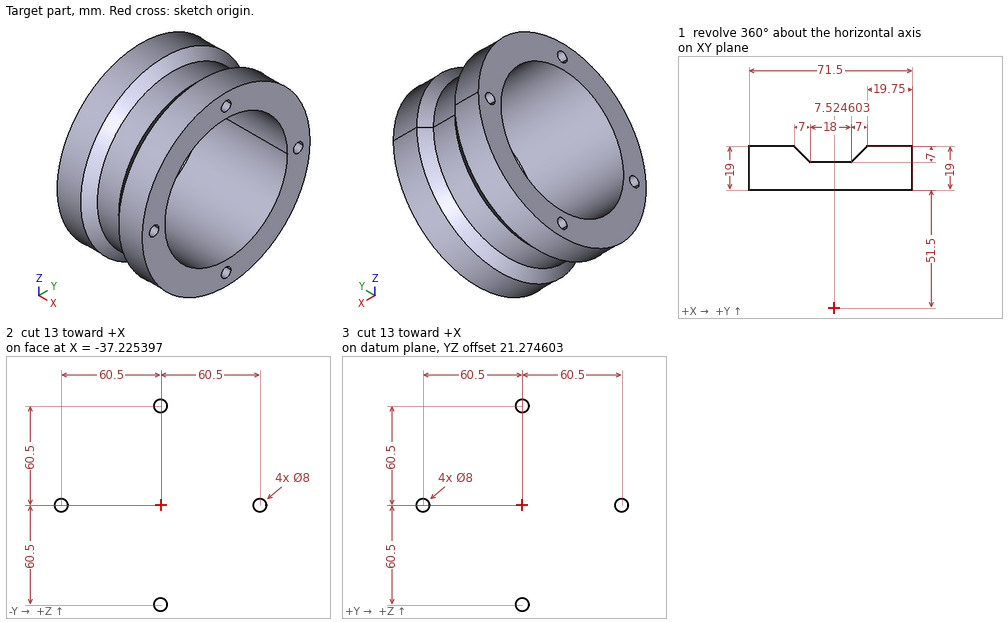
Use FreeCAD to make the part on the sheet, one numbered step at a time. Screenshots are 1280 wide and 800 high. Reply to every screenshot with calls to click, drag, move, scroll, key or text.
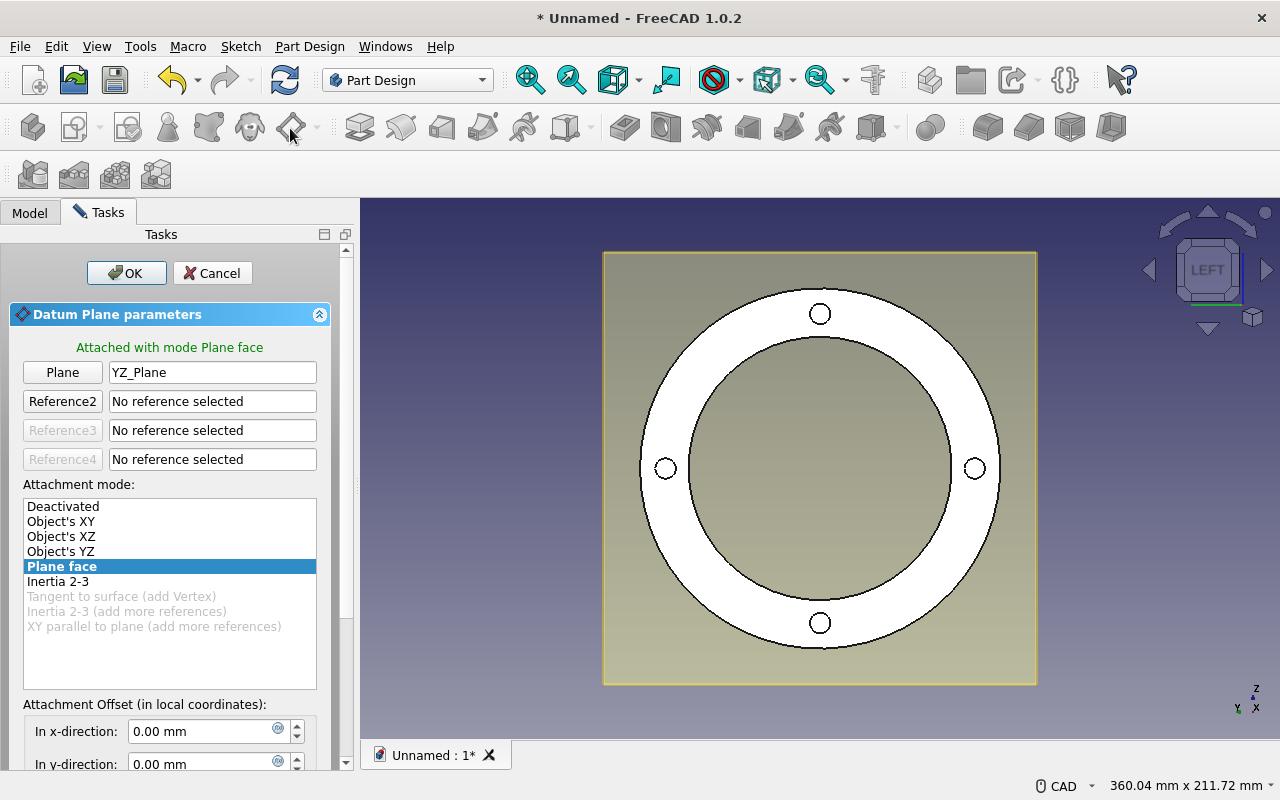
scroll(346, 507, down, 2)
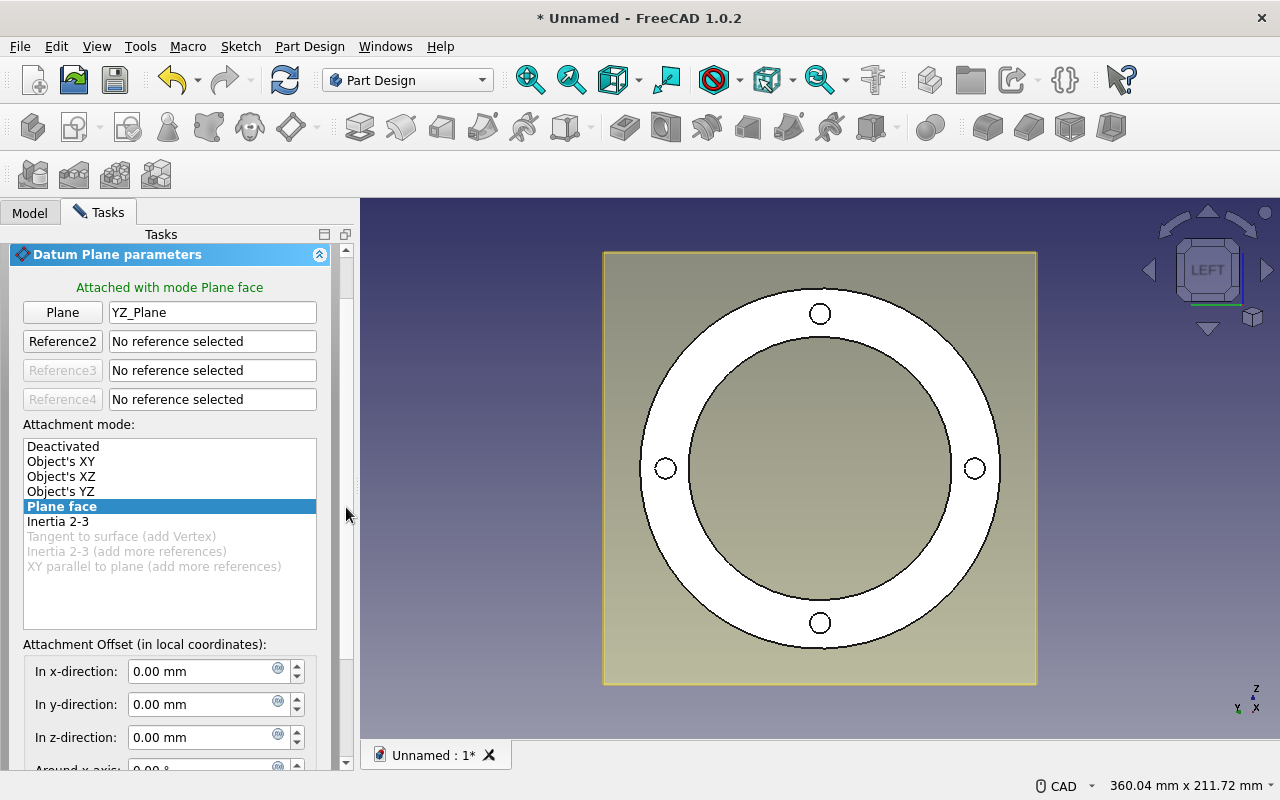
triple_click(210, 678)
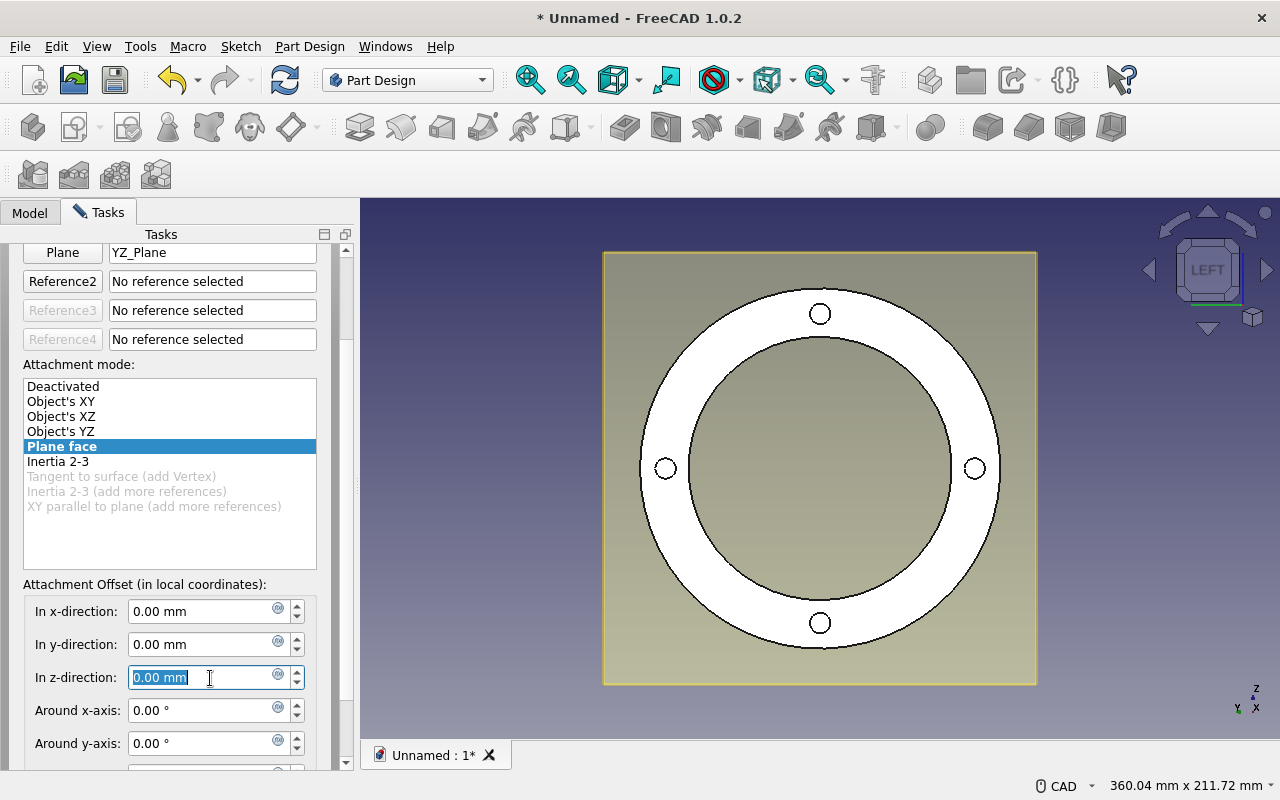
text(21.274603)
key(Tab)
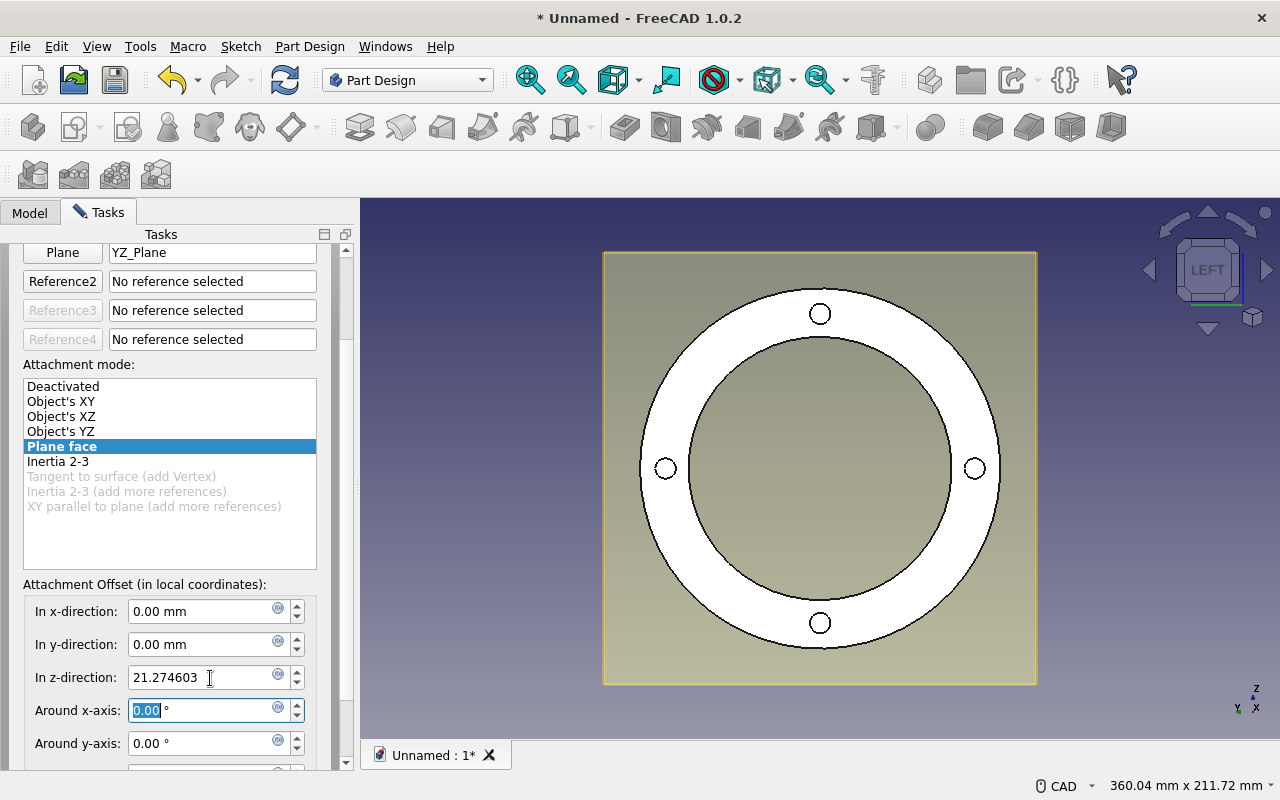
scroll(346, 507, up, 3)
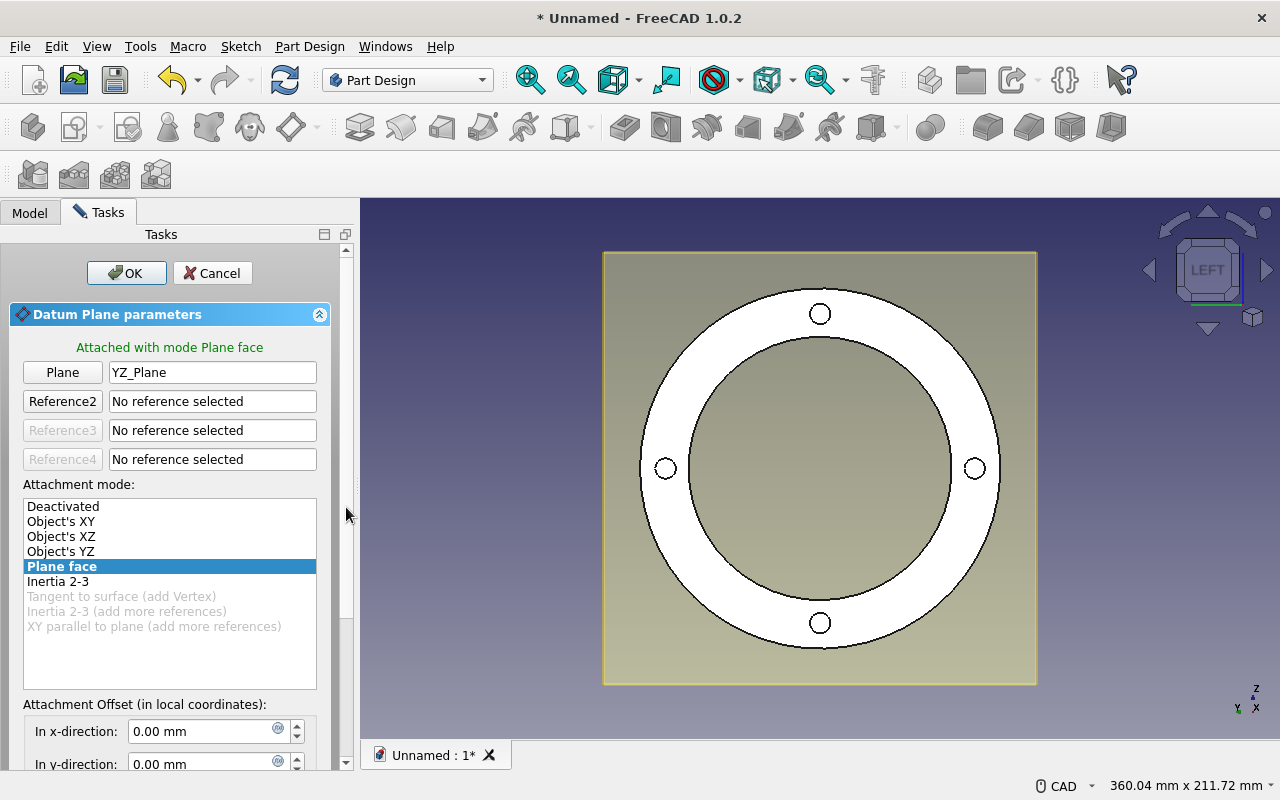
click(127, 273)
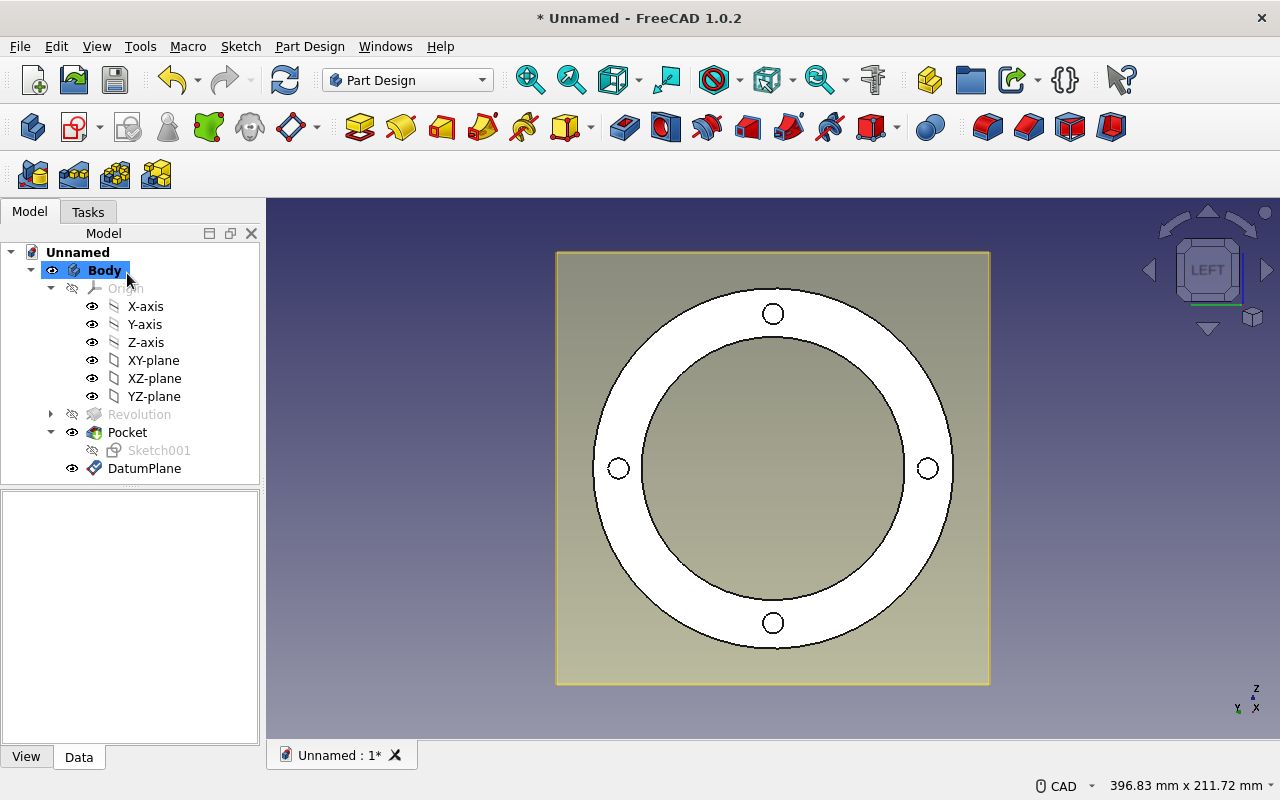
click(117, 468)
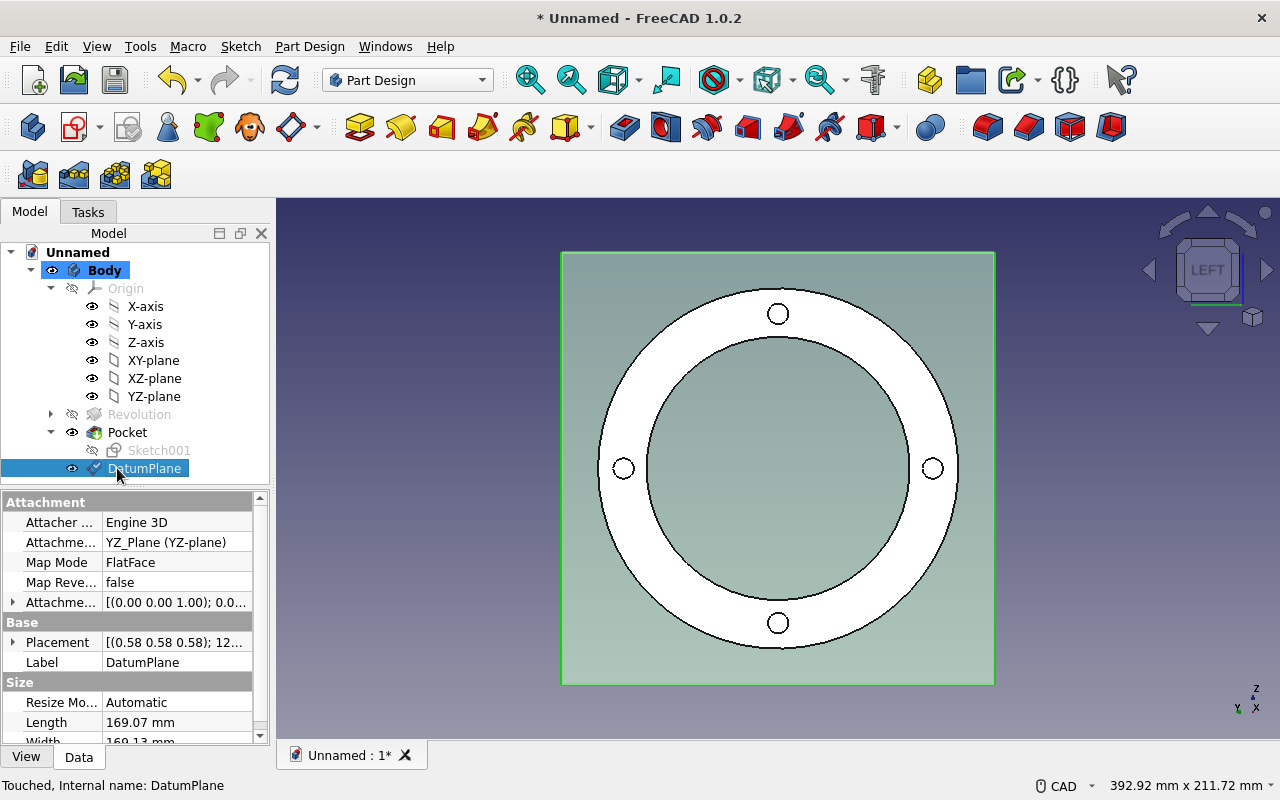
click(74, 128)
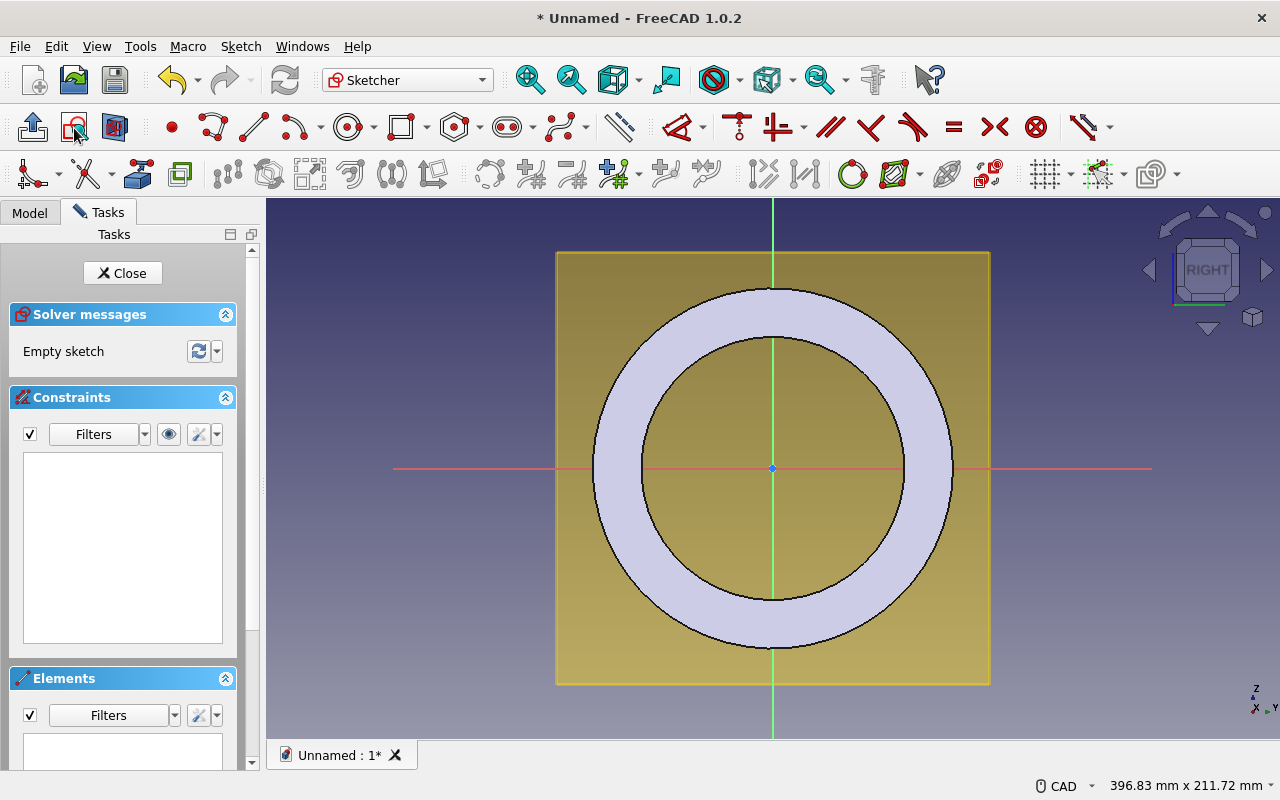
click(115, 128)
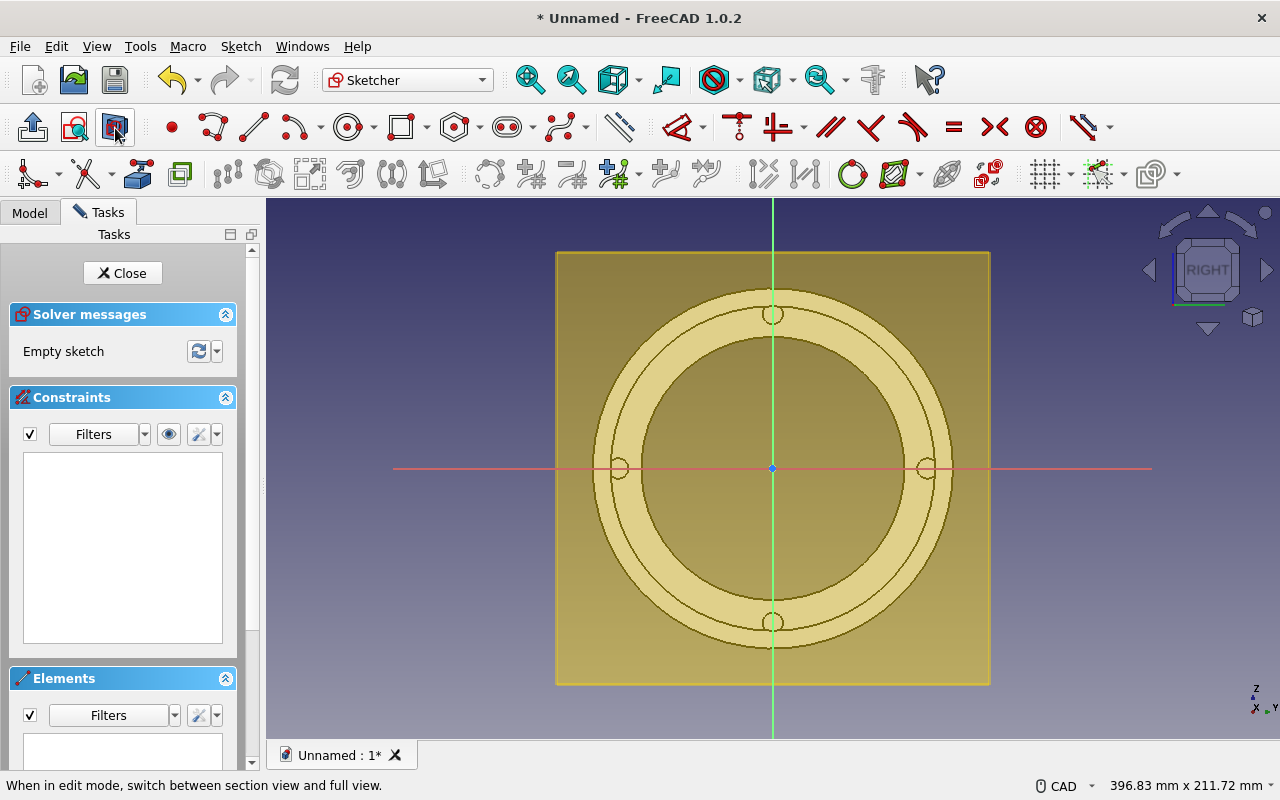
click(348, 128)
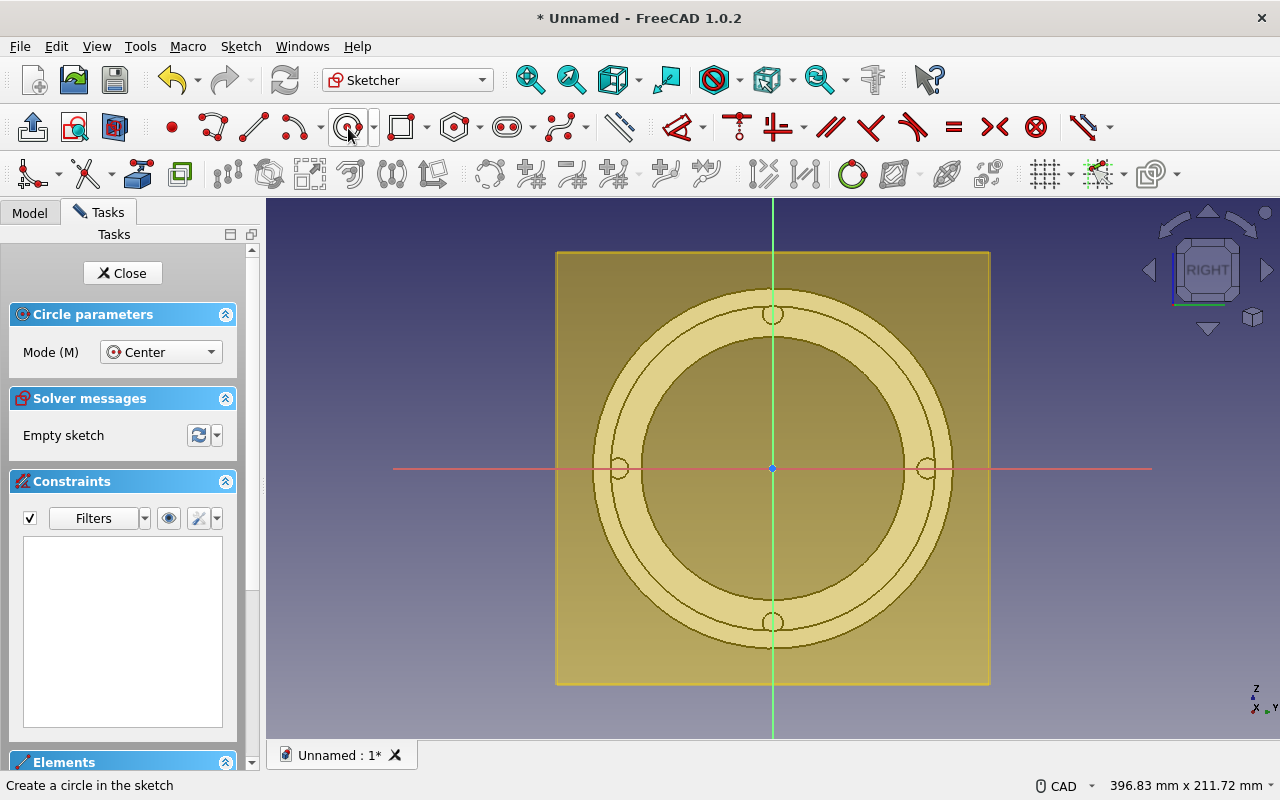
scroll(618, 469, up, 4)